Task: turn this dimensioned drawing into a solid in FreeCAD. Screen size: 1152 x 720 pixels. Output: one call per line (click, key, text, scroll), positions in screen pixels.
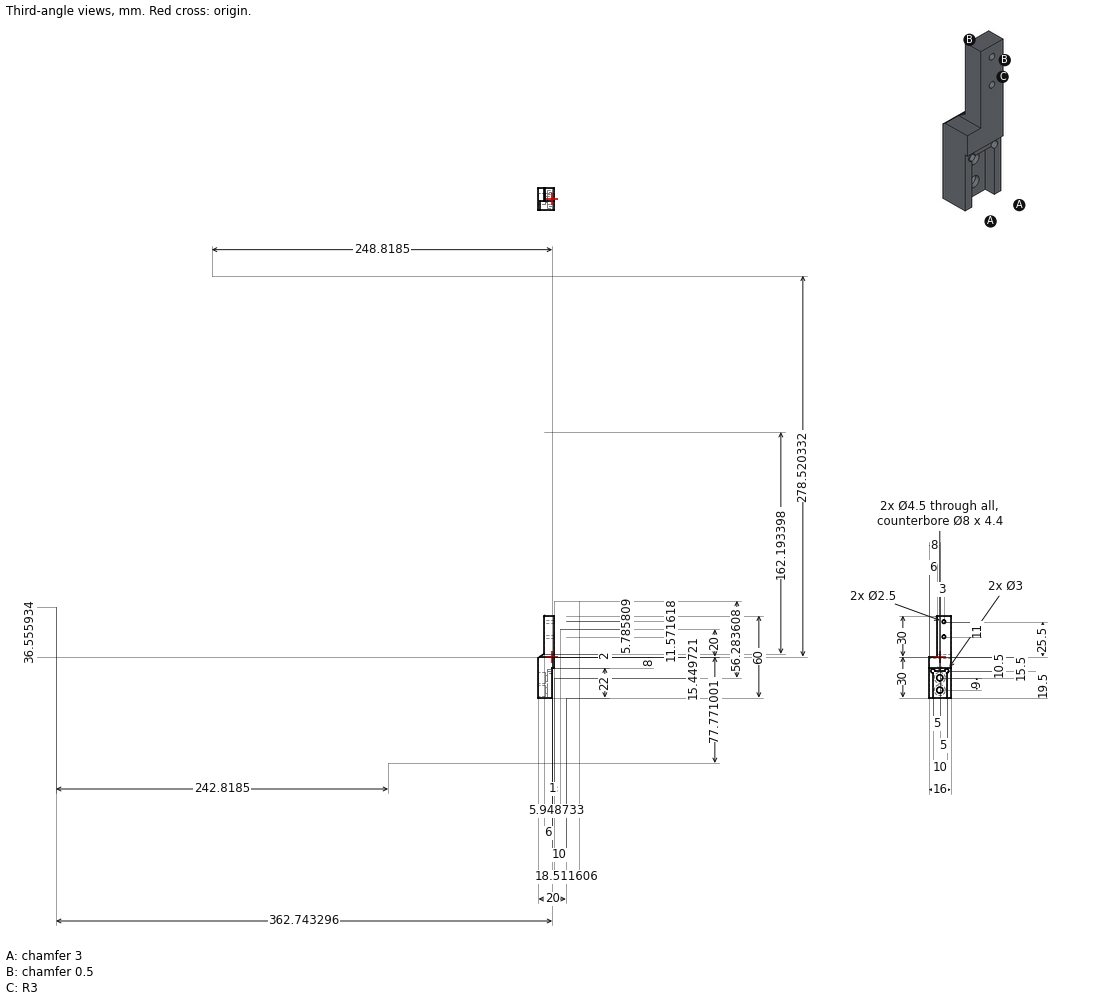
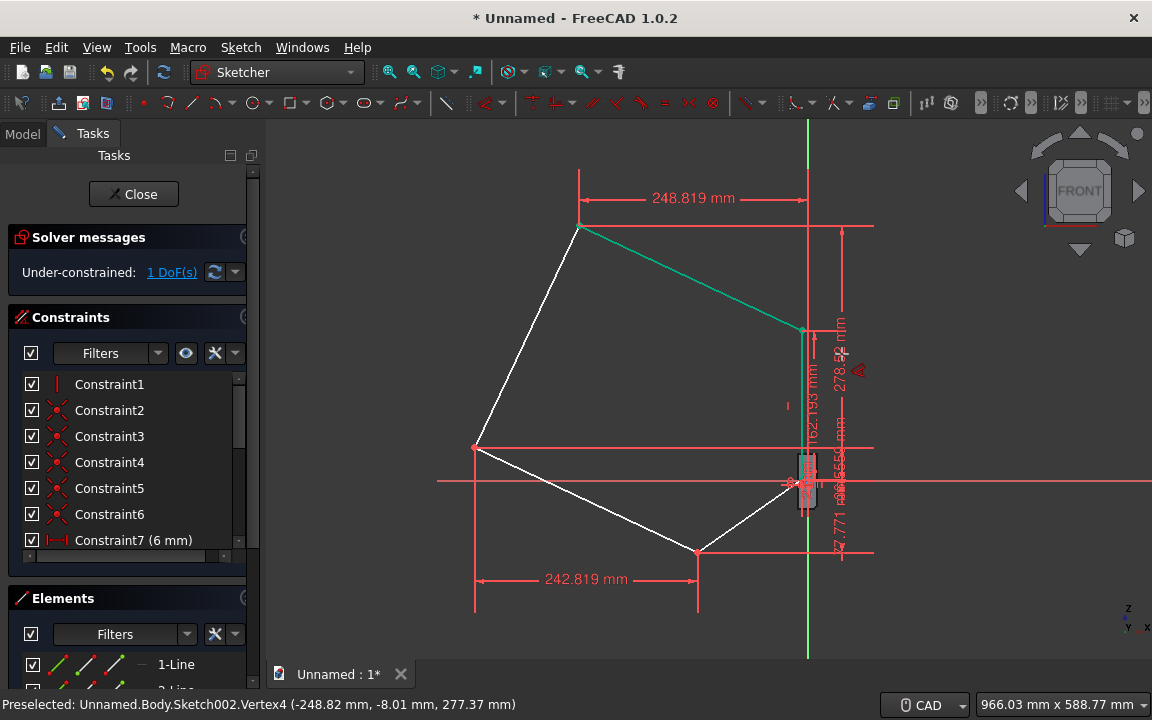
click(475, 448)
click(565, 515)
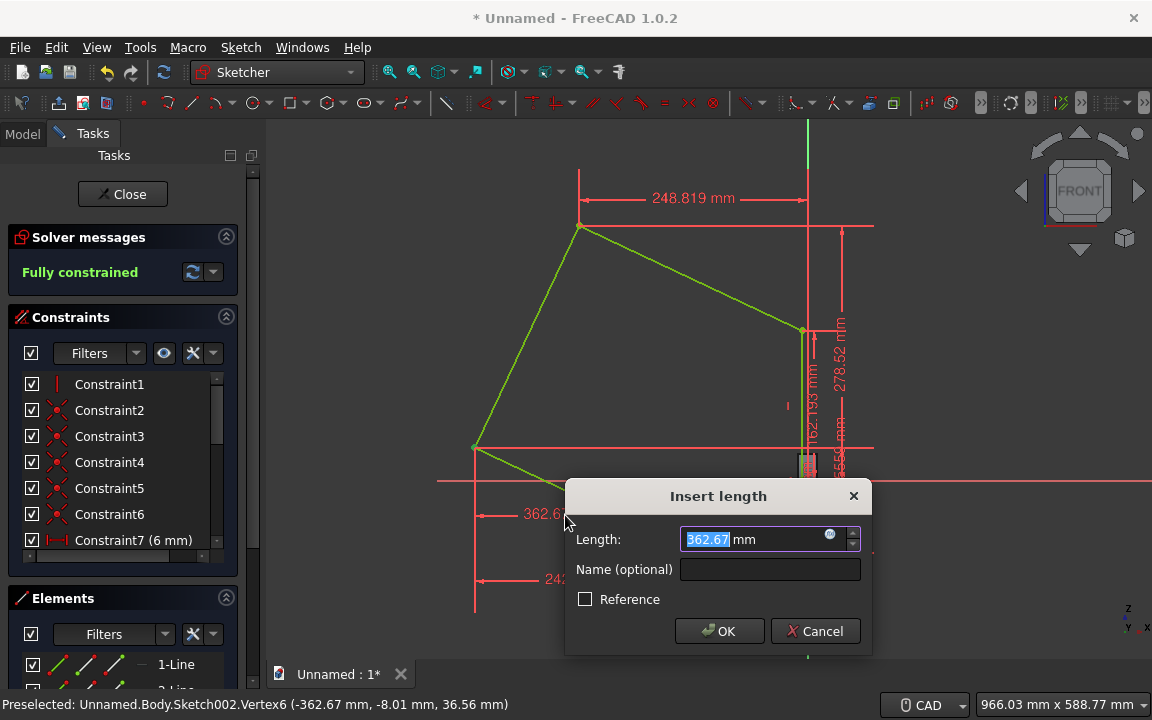
text(362.743296)
key(Return)
key(Escape)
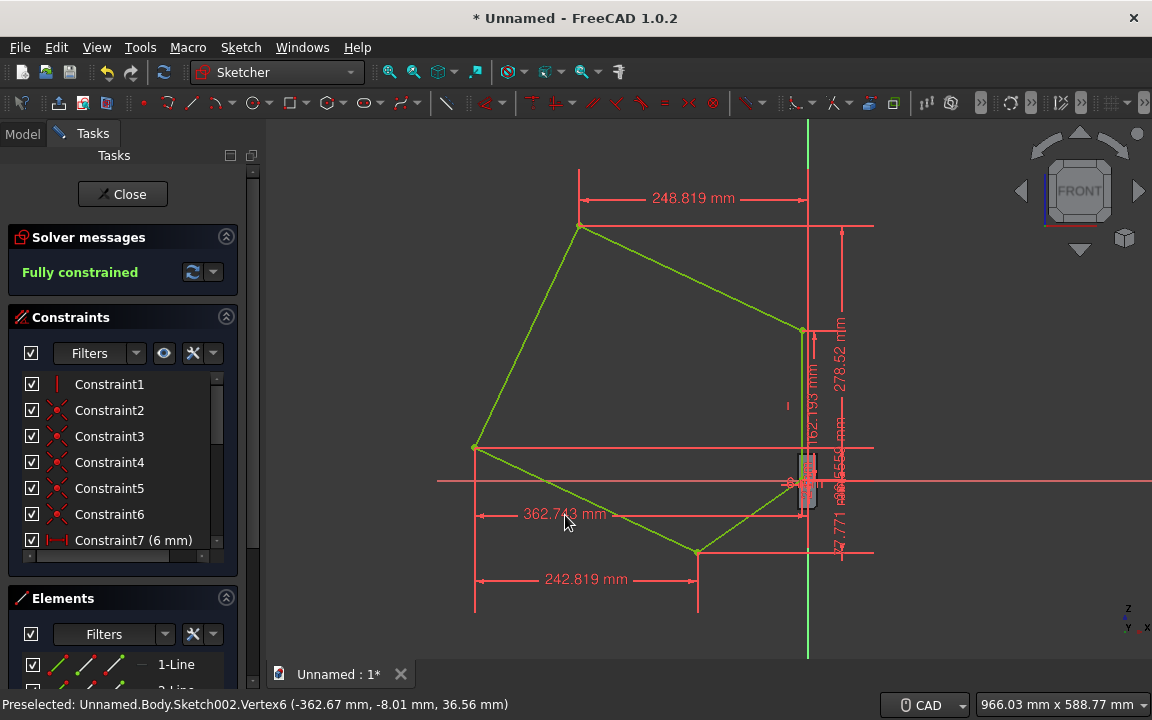
click(123, 194)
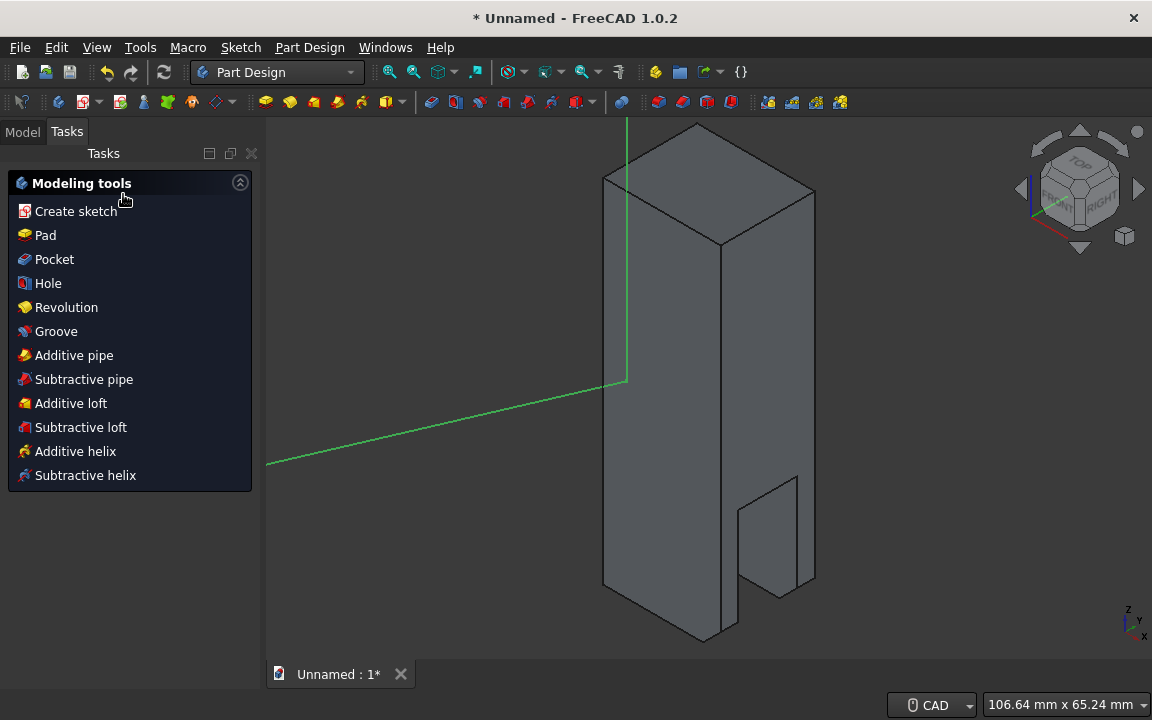
click(432, 102)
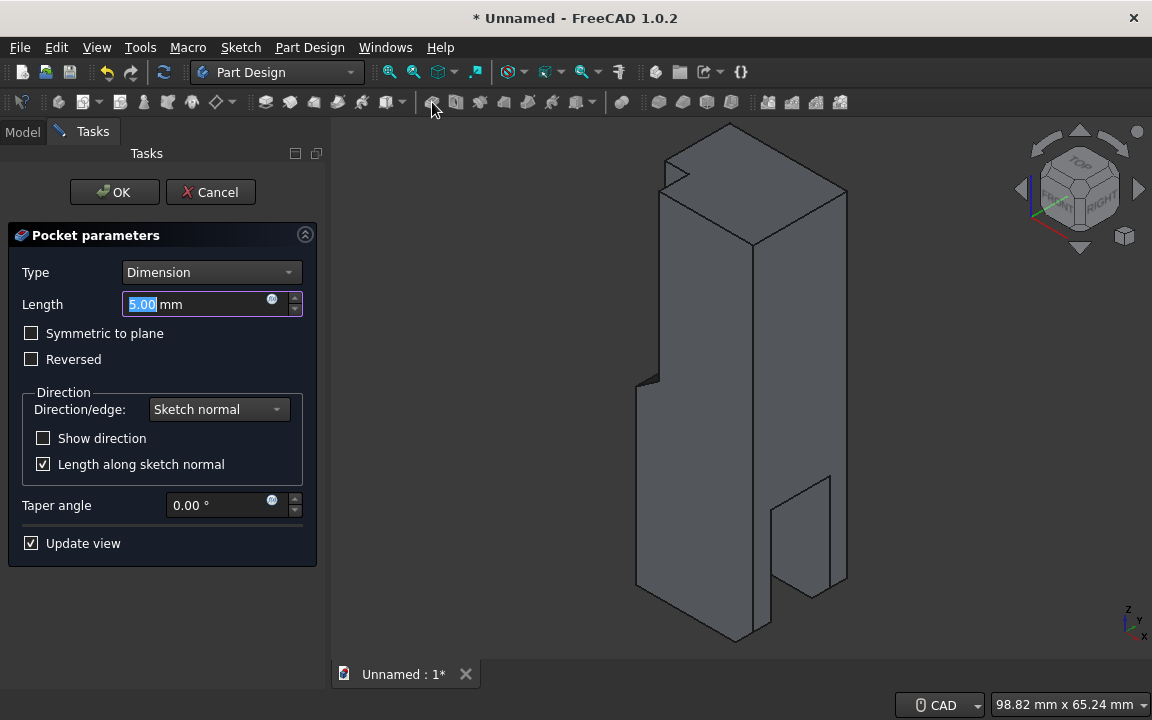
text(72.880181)
key(Tab)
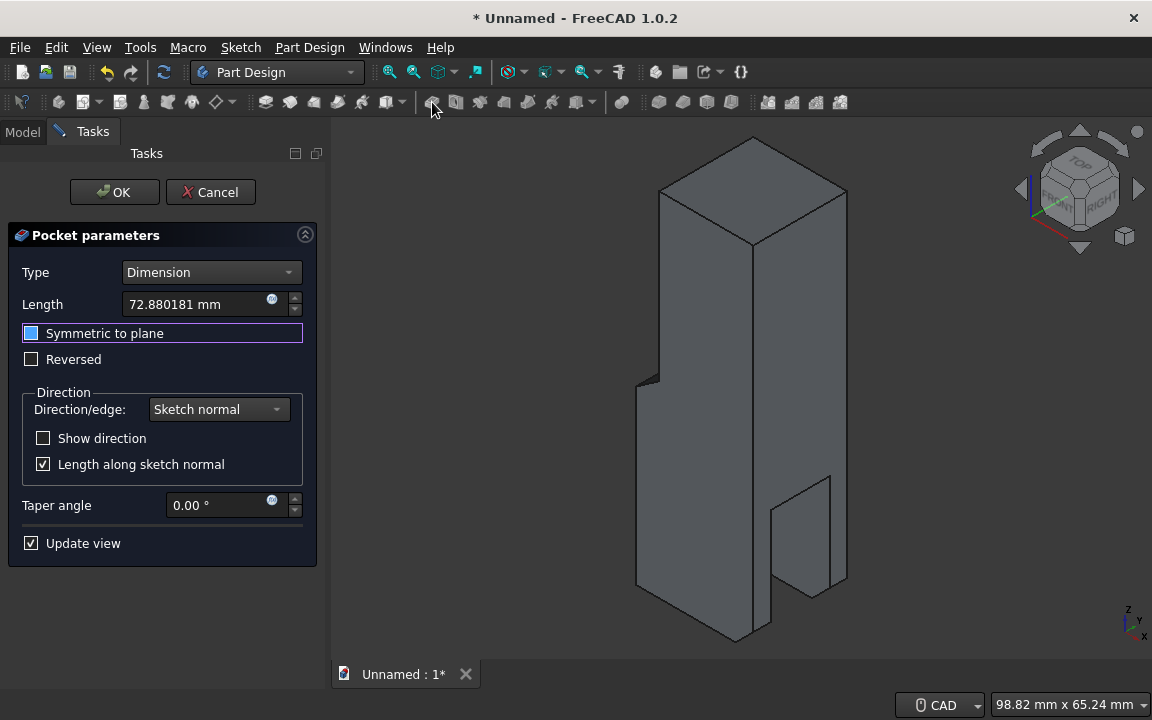
click(30, 333)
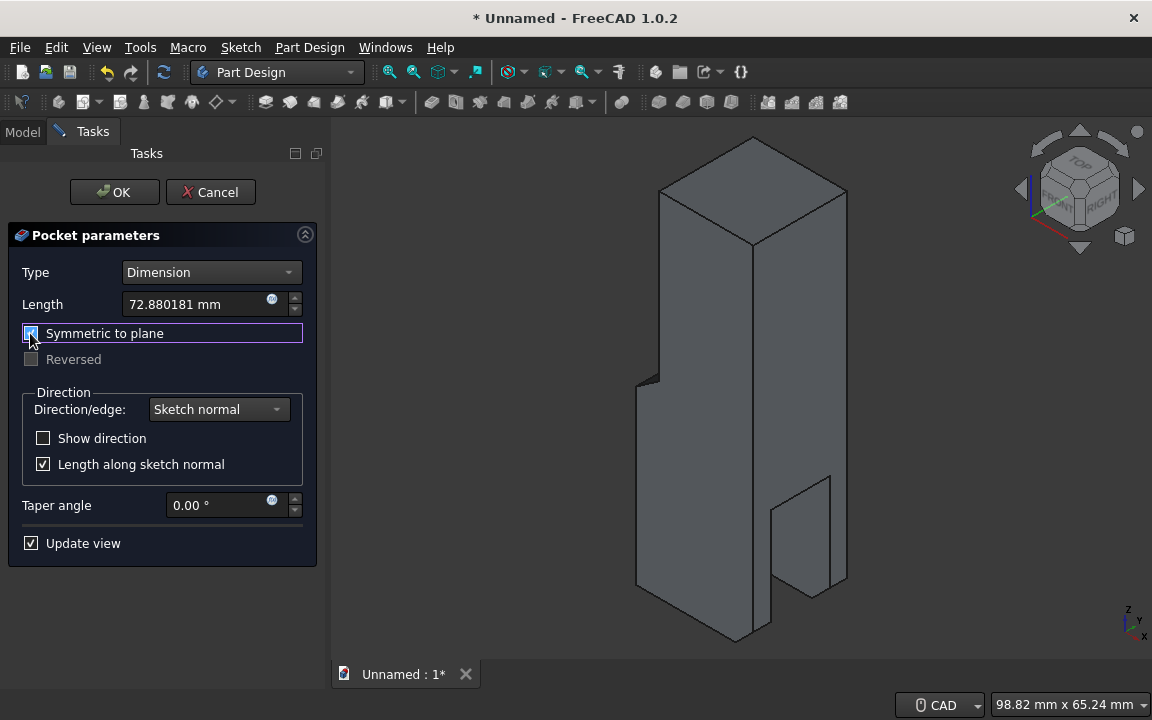
click(115, 192)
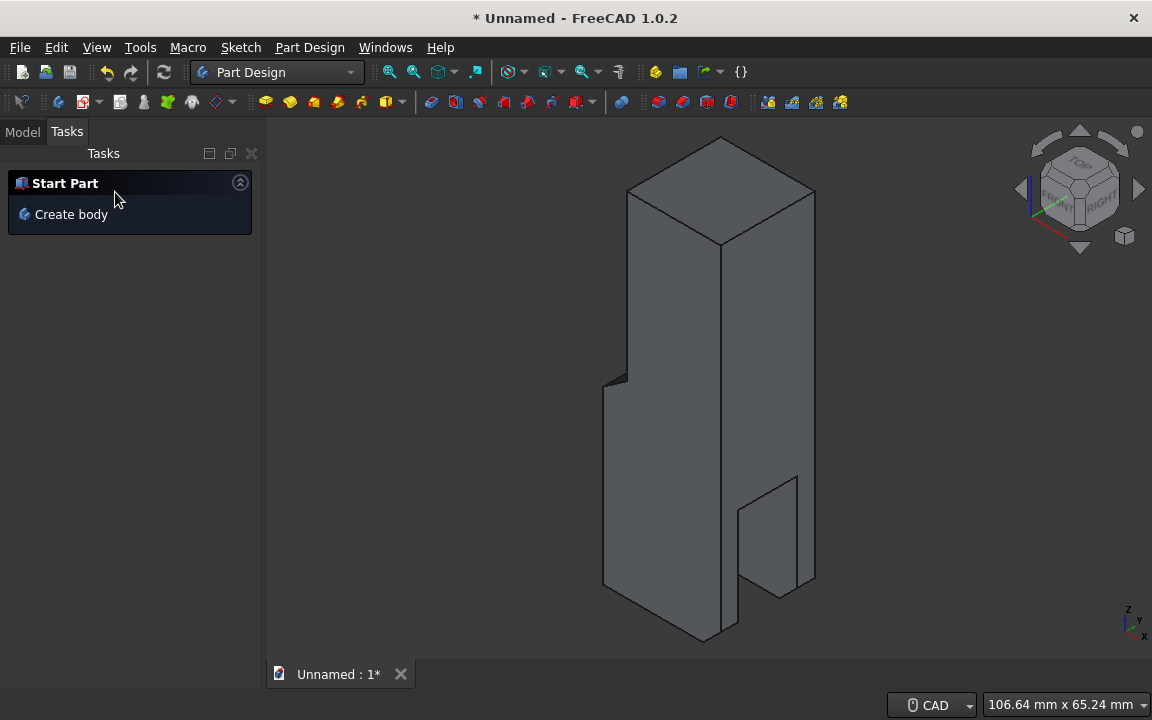
click(768, 217)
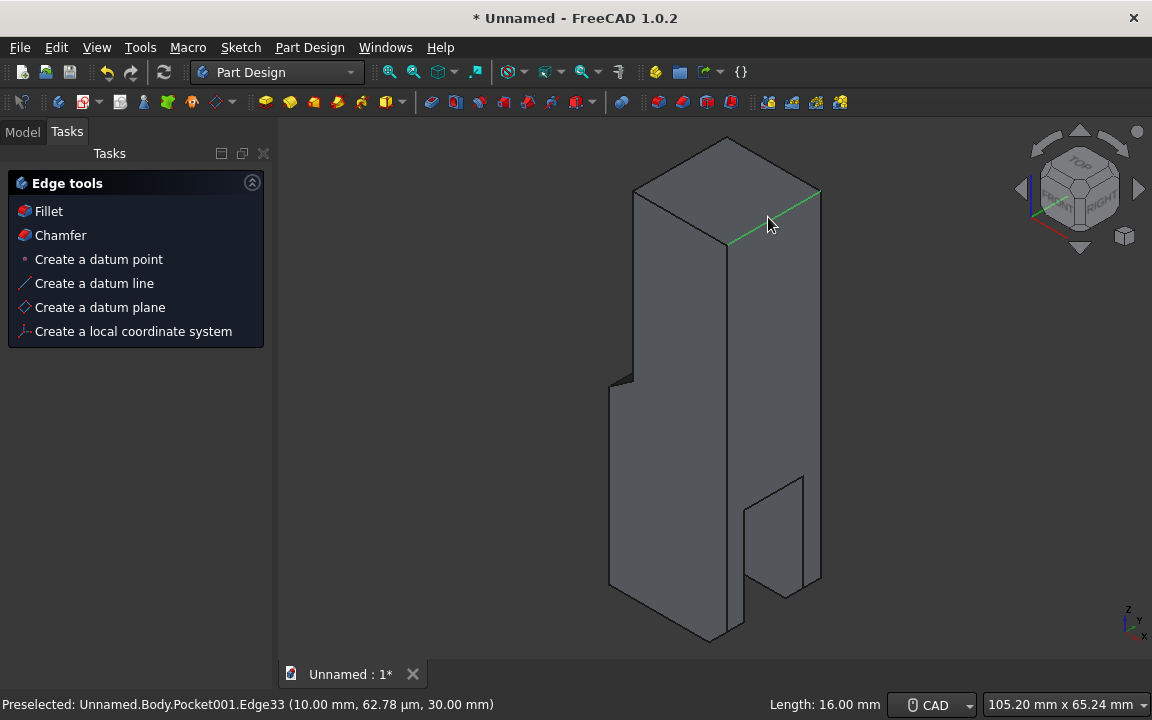
key(2)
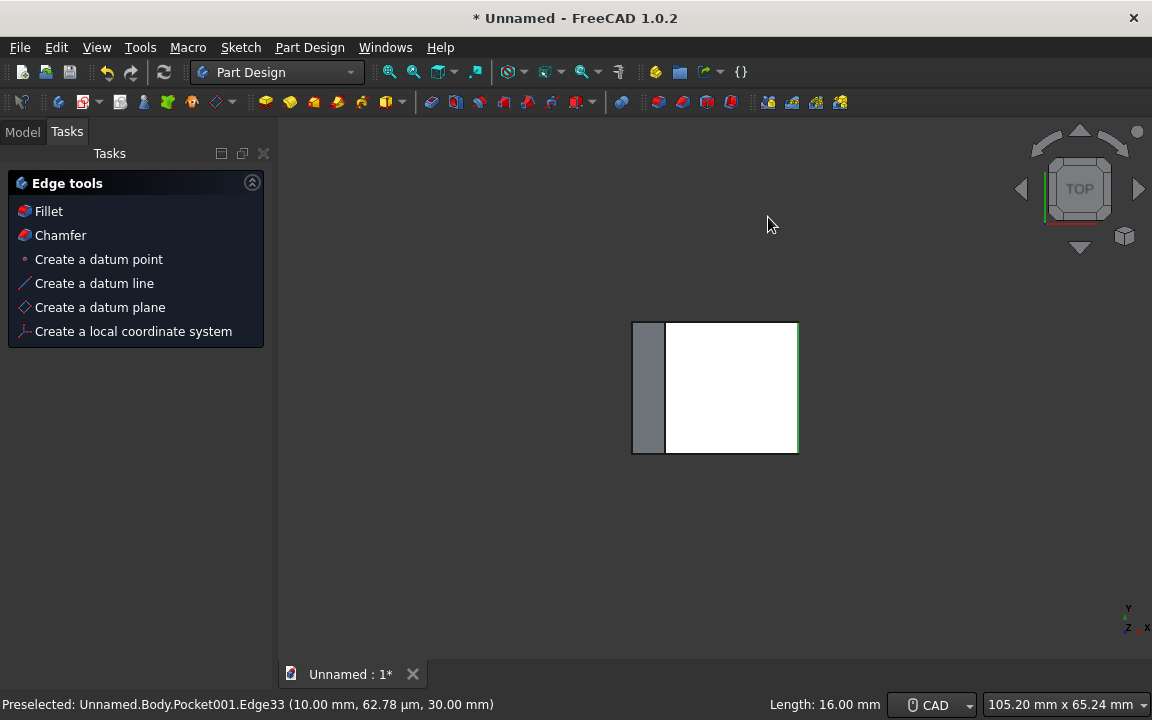
click(390, 72)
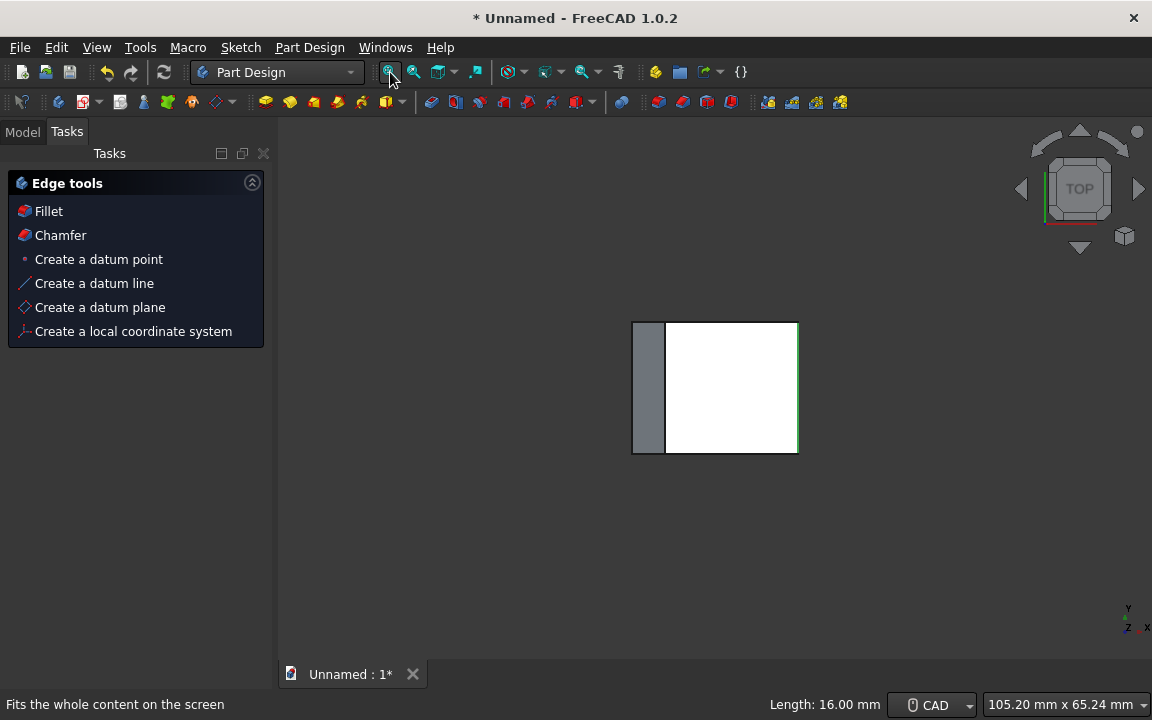
click(665, 387, ctrl)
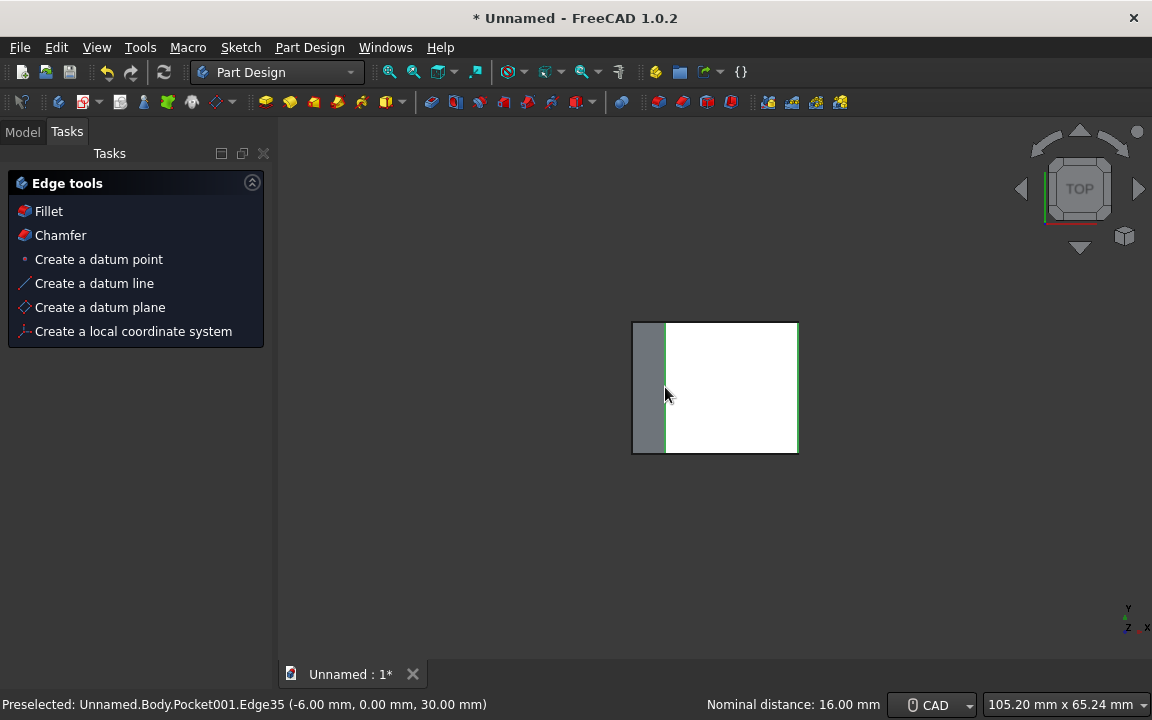
click(684, 102)